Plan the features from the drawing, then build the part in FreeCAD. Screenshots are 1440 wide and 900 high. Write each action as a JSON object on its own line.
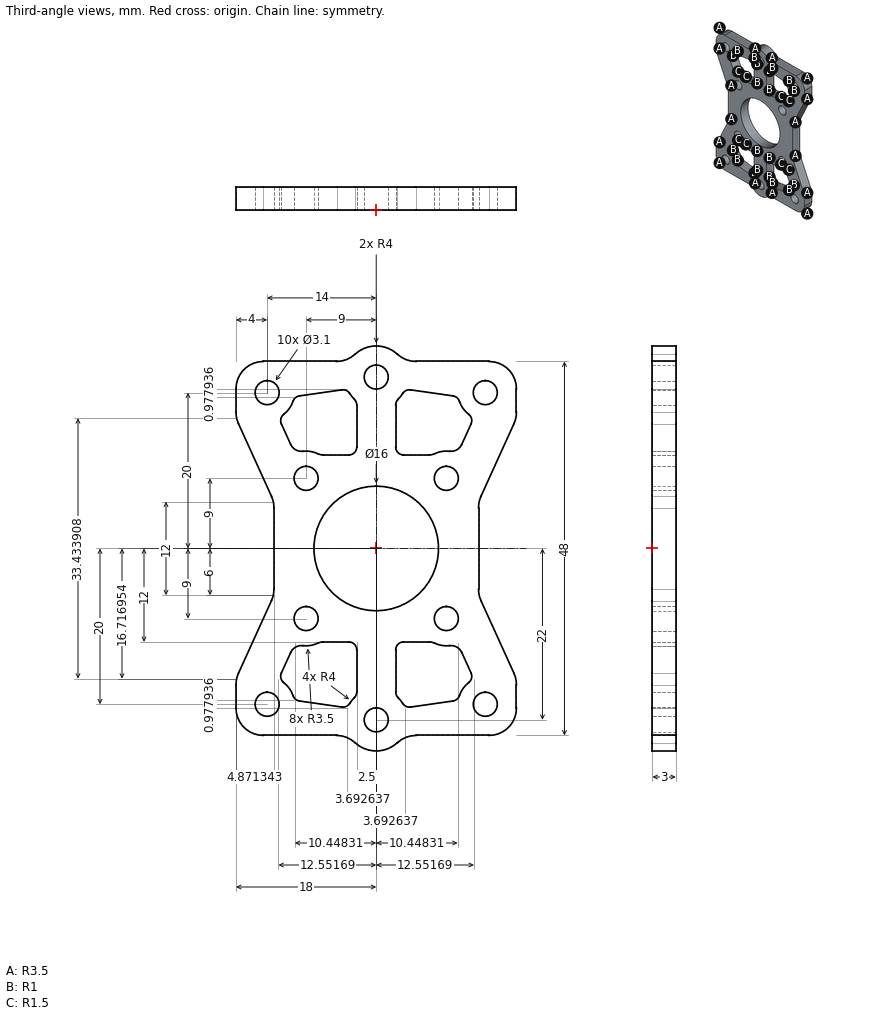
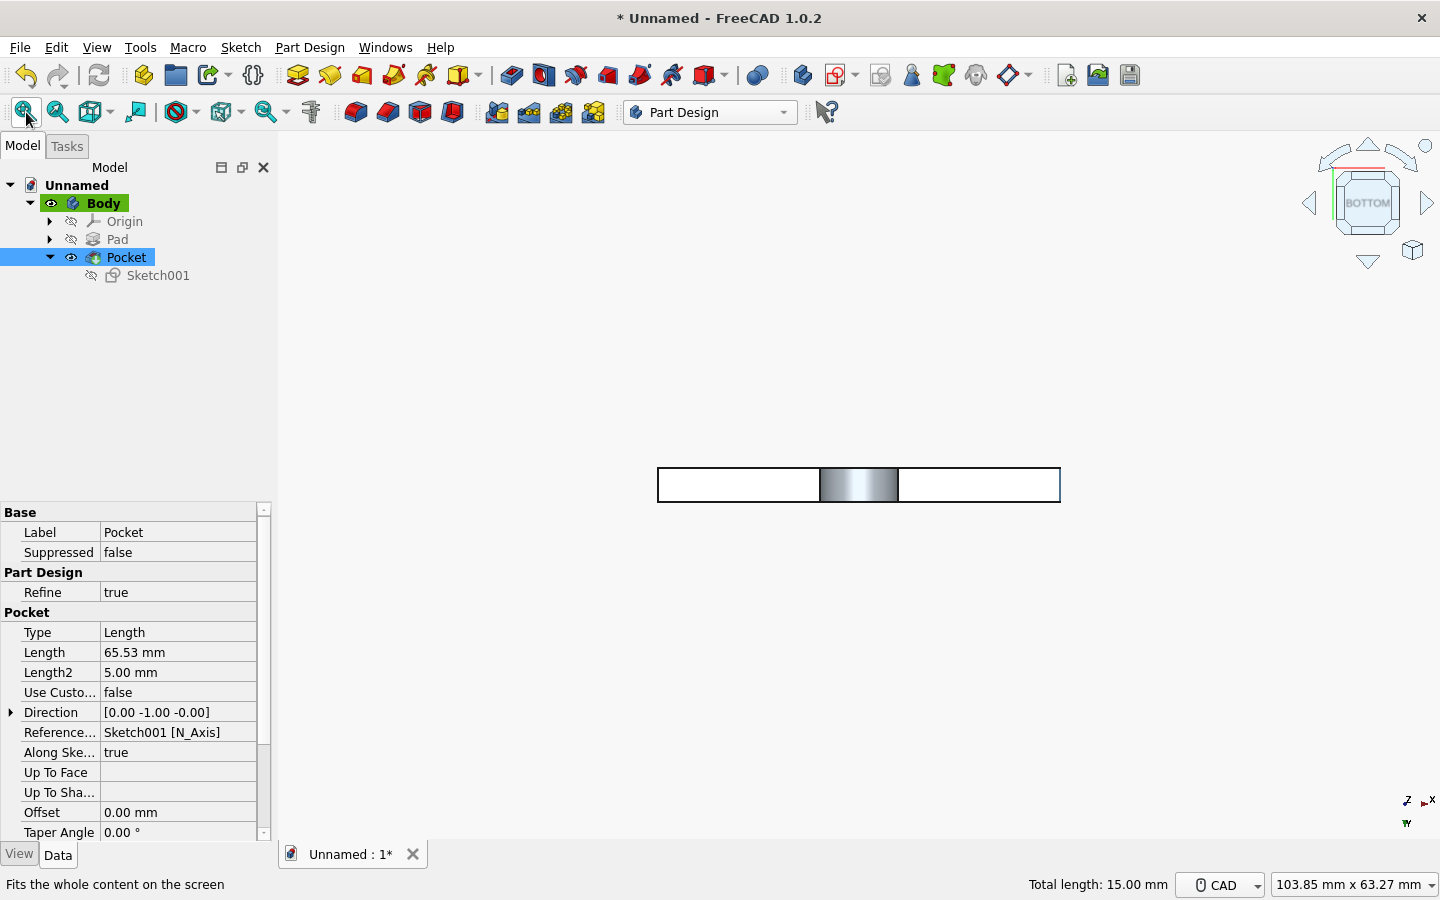
{"action": "left_click", "coordinate": [658, 484], "text": "ctrl"}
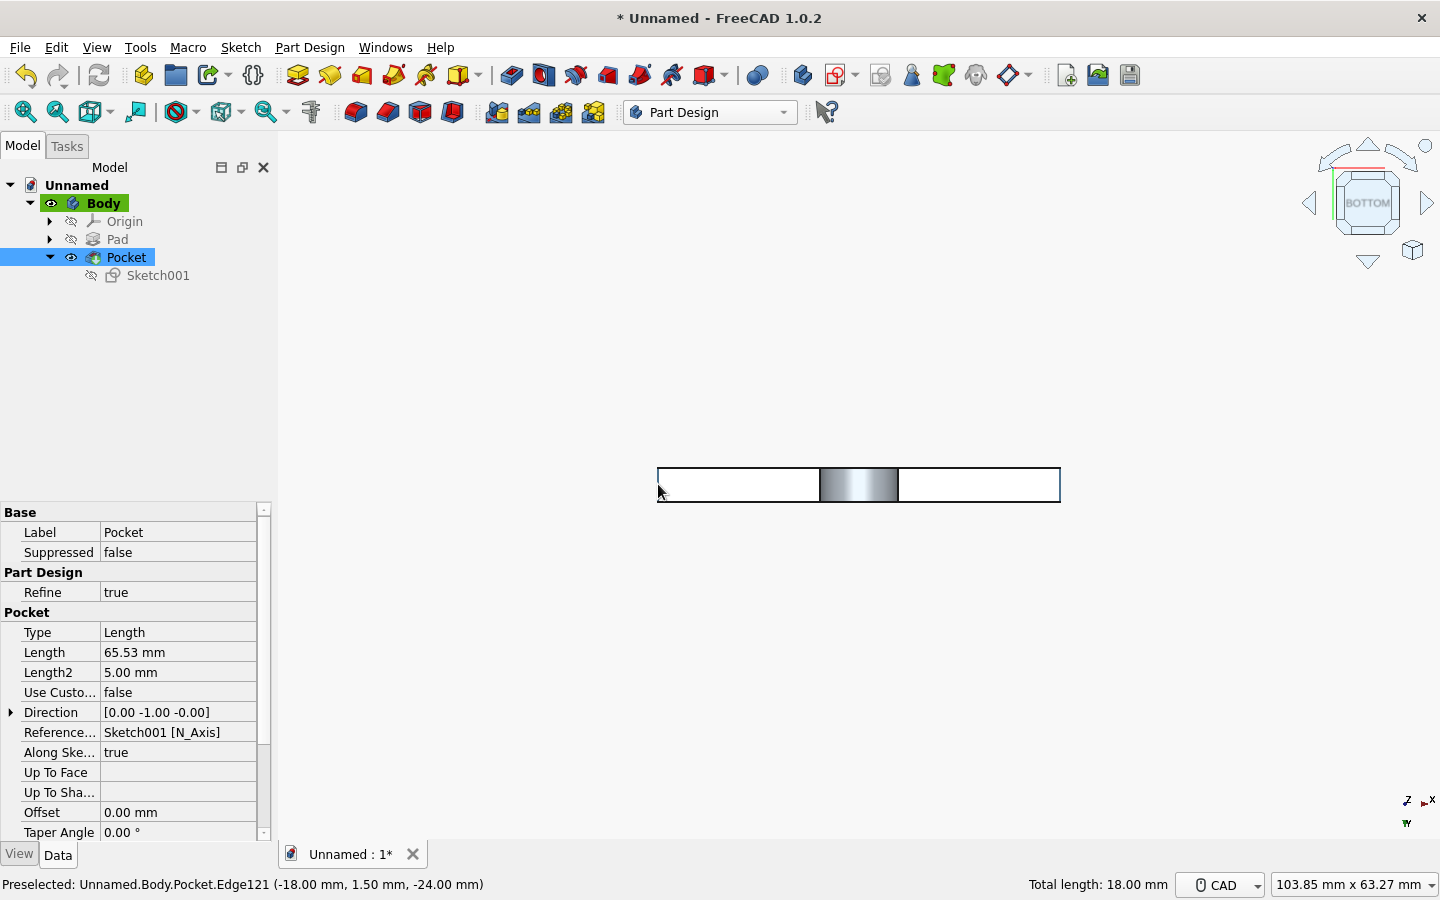
{"action": "key", "text": "4"}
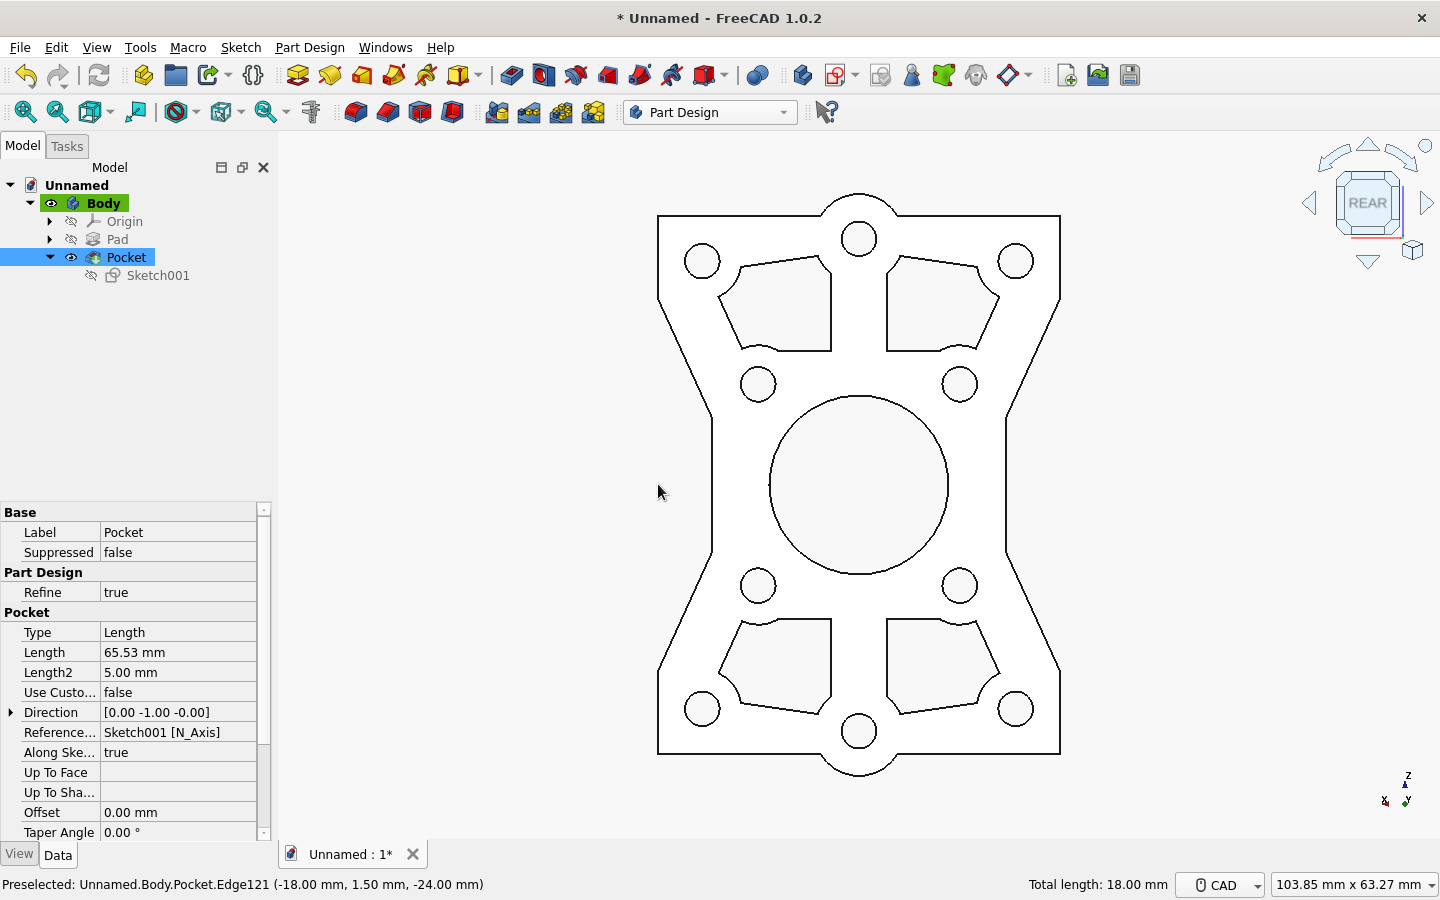
{"action": "key", "text": "6"}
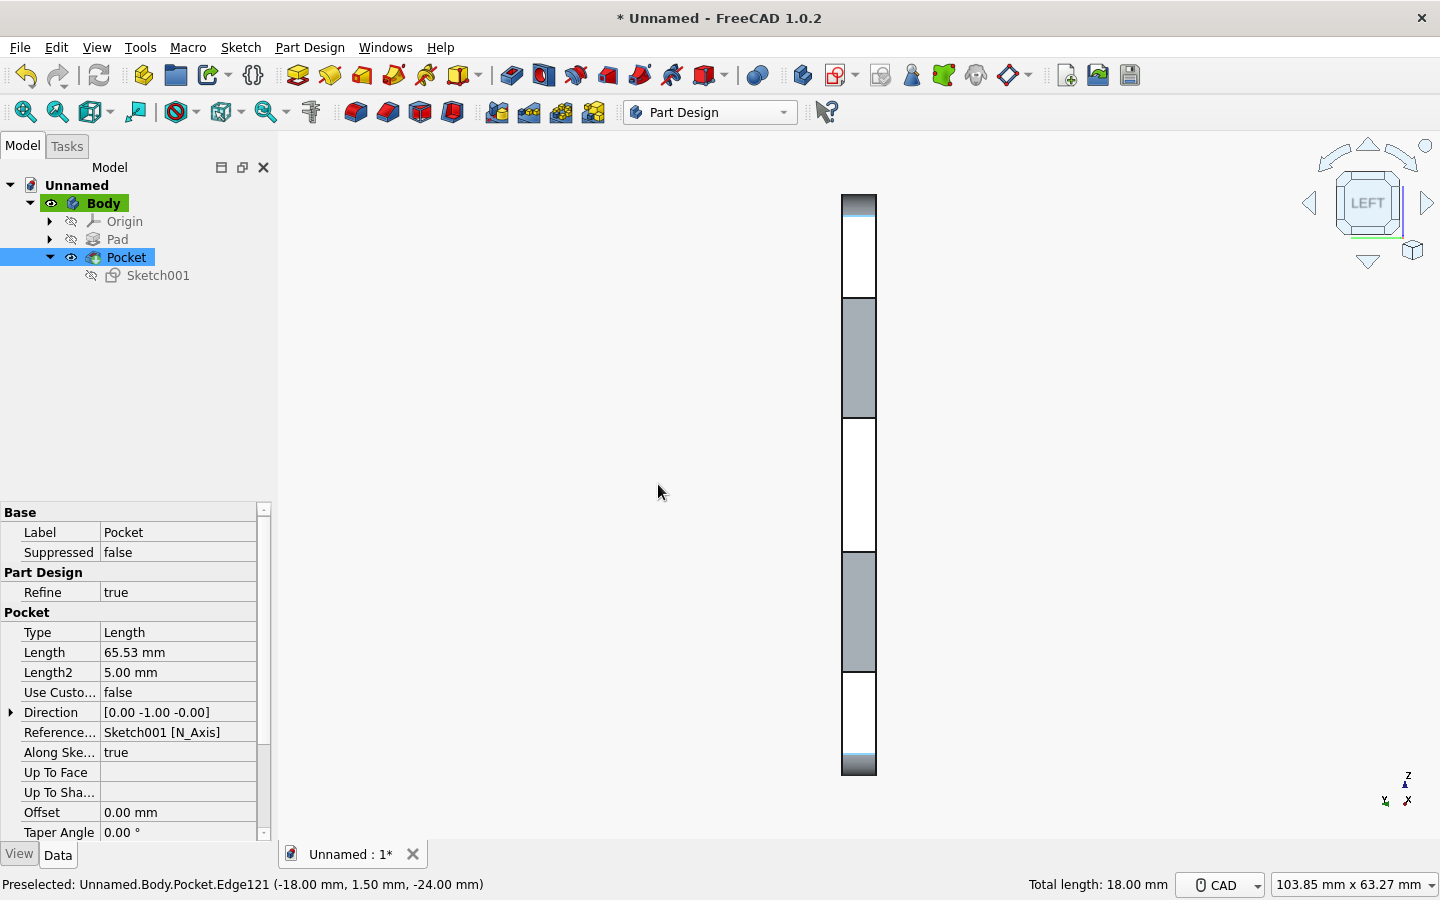
{"action": "left_click", "coordinate": [859, 671], "text": "ctrl"}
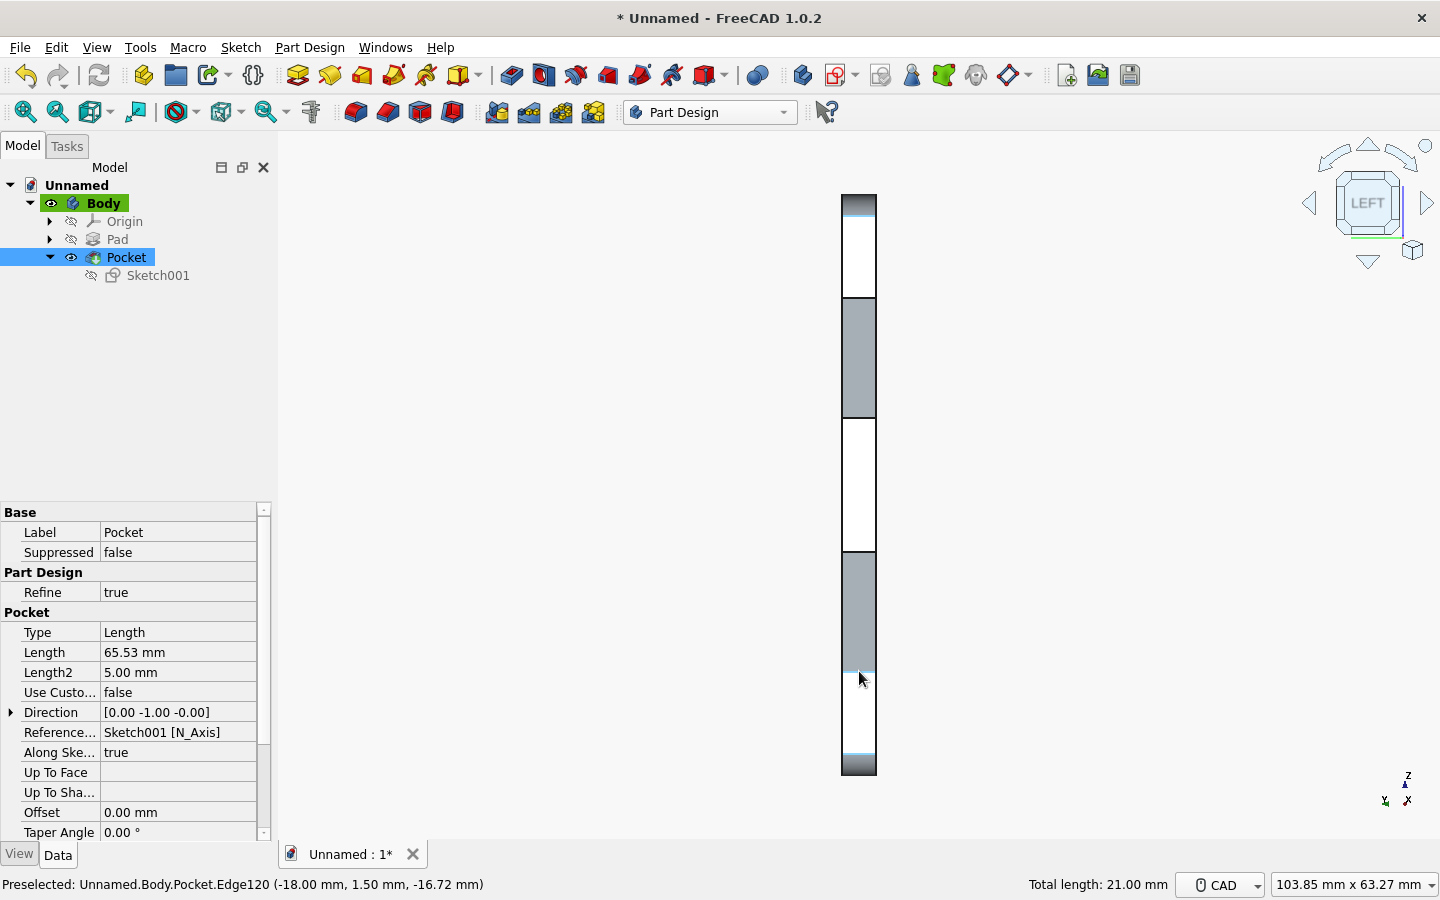
{"action": "left_click", "coordinate": [859, 297], "text": "ctrl"}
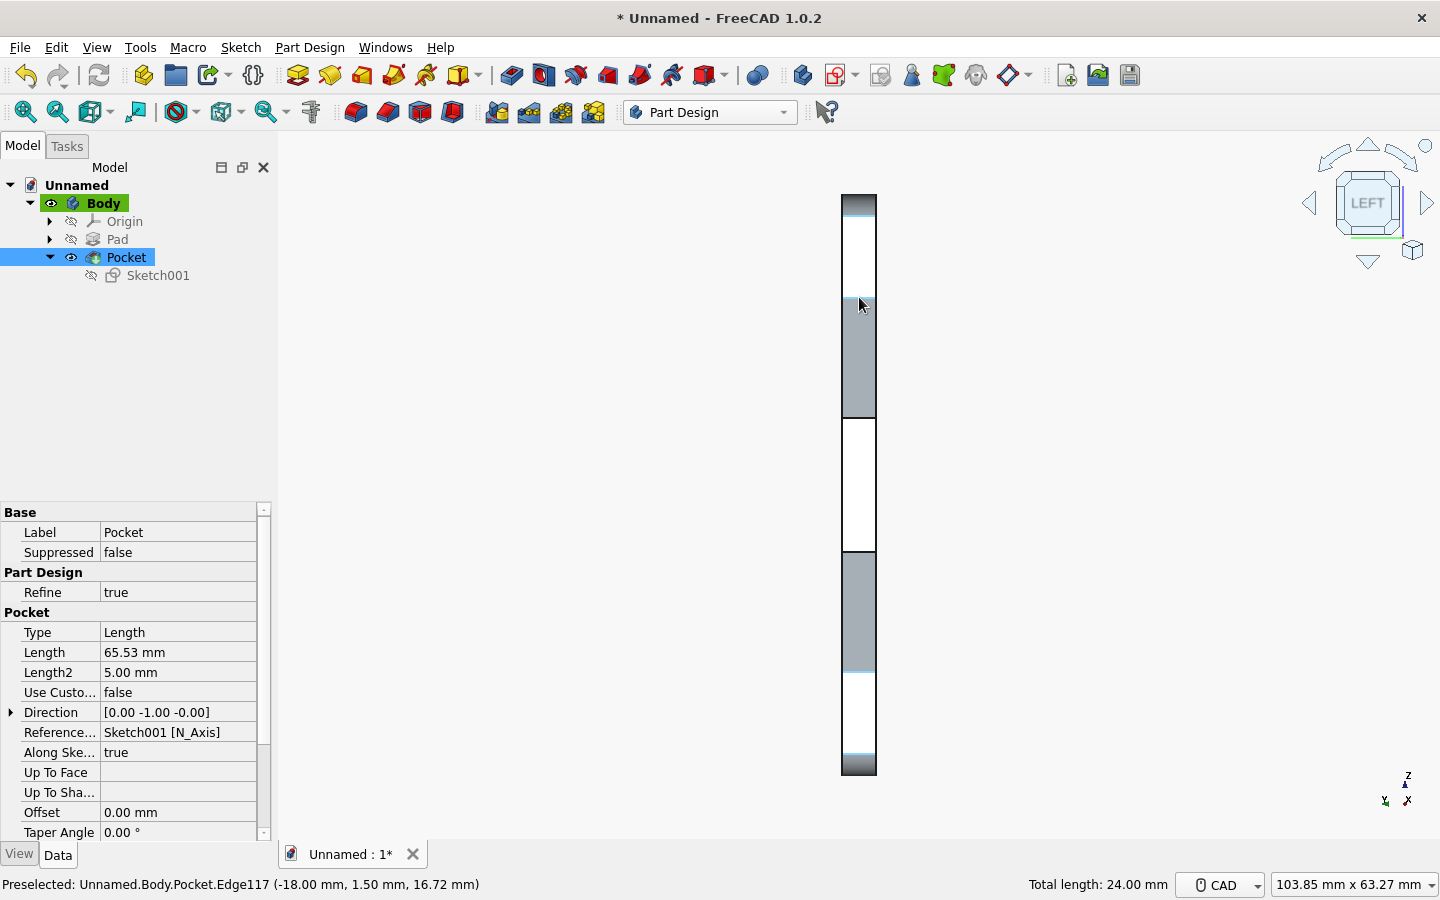
{"action": "key", "text": "v 3"}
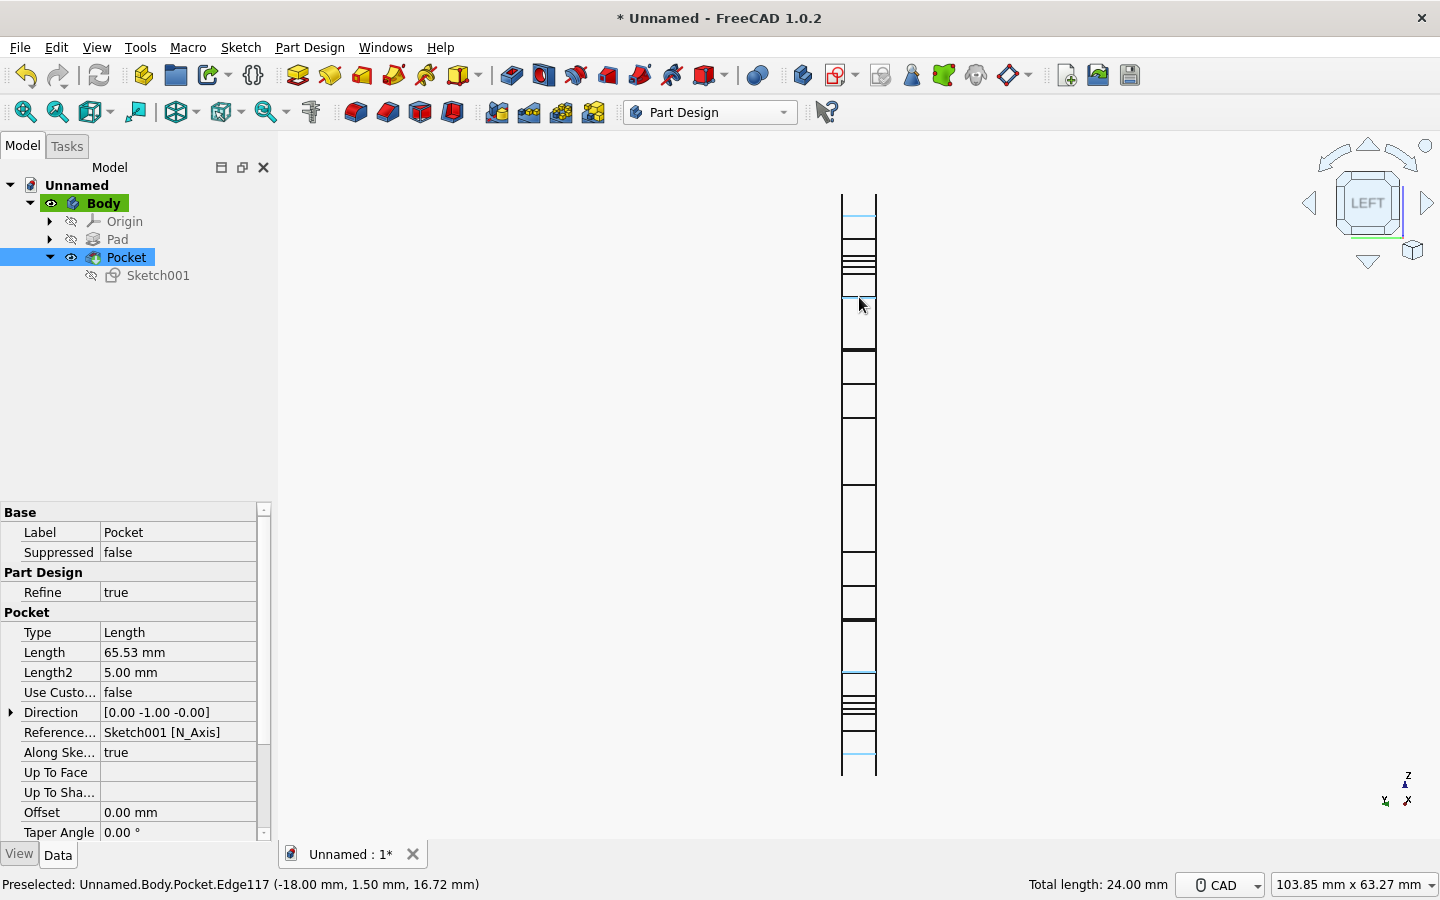
{"action": "key", "text": "0"}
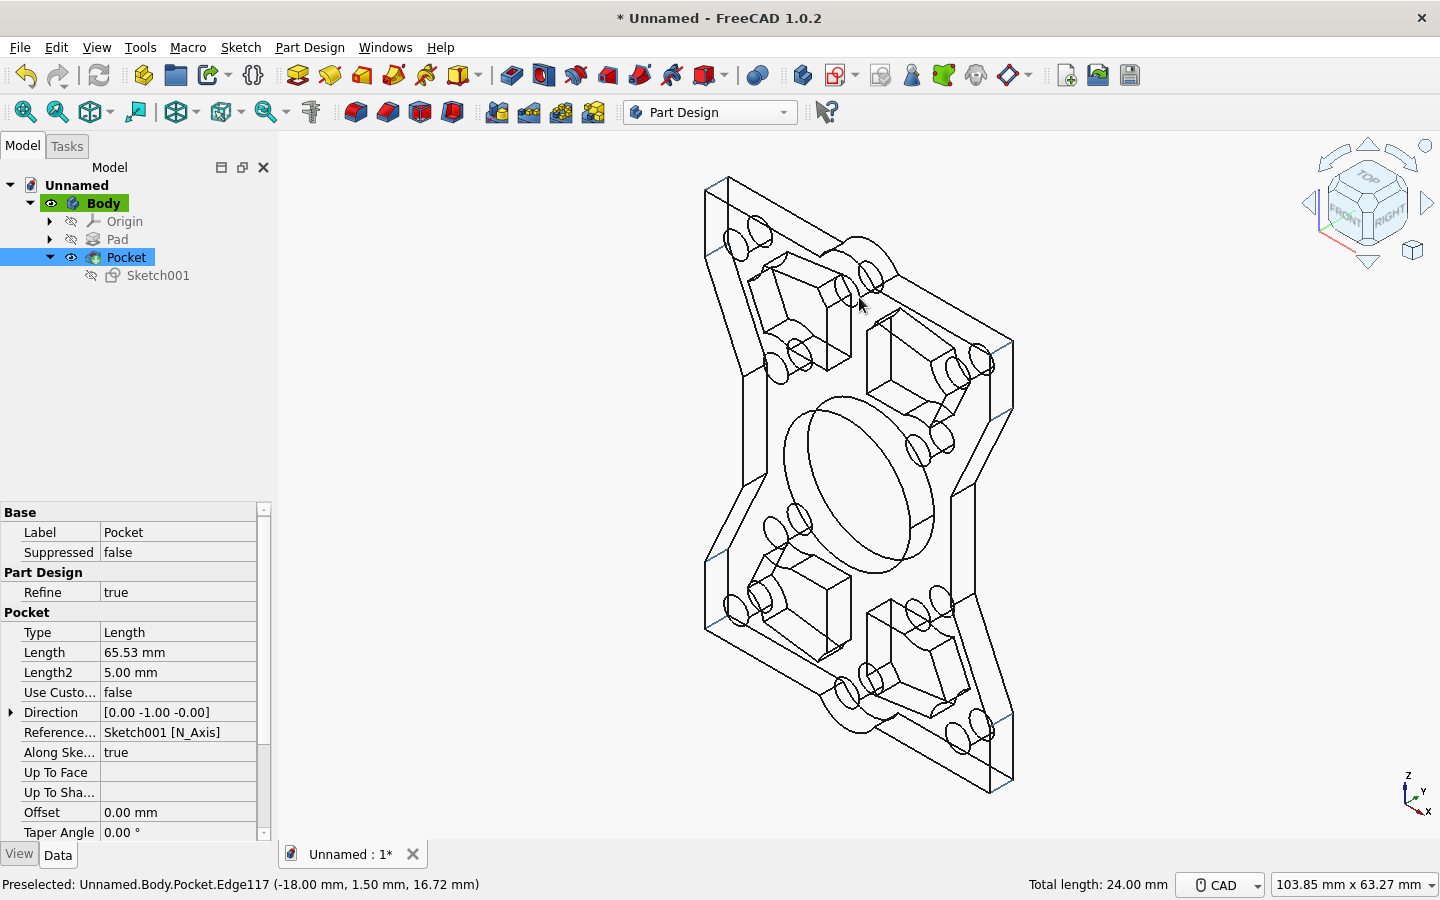
{"action": "left_click", "coordinate": [963, 489], "text": "ctrl"}